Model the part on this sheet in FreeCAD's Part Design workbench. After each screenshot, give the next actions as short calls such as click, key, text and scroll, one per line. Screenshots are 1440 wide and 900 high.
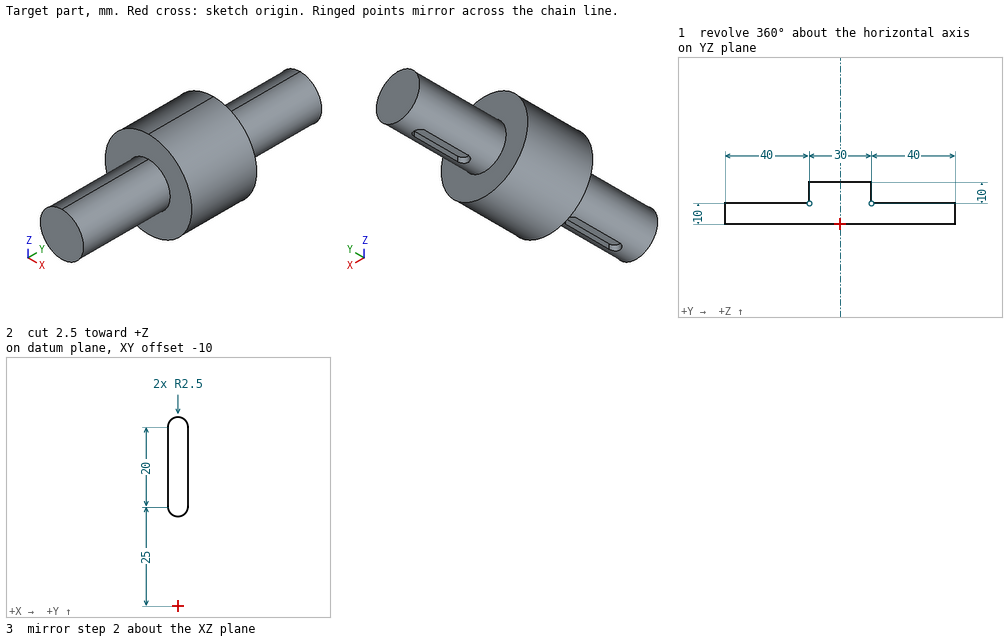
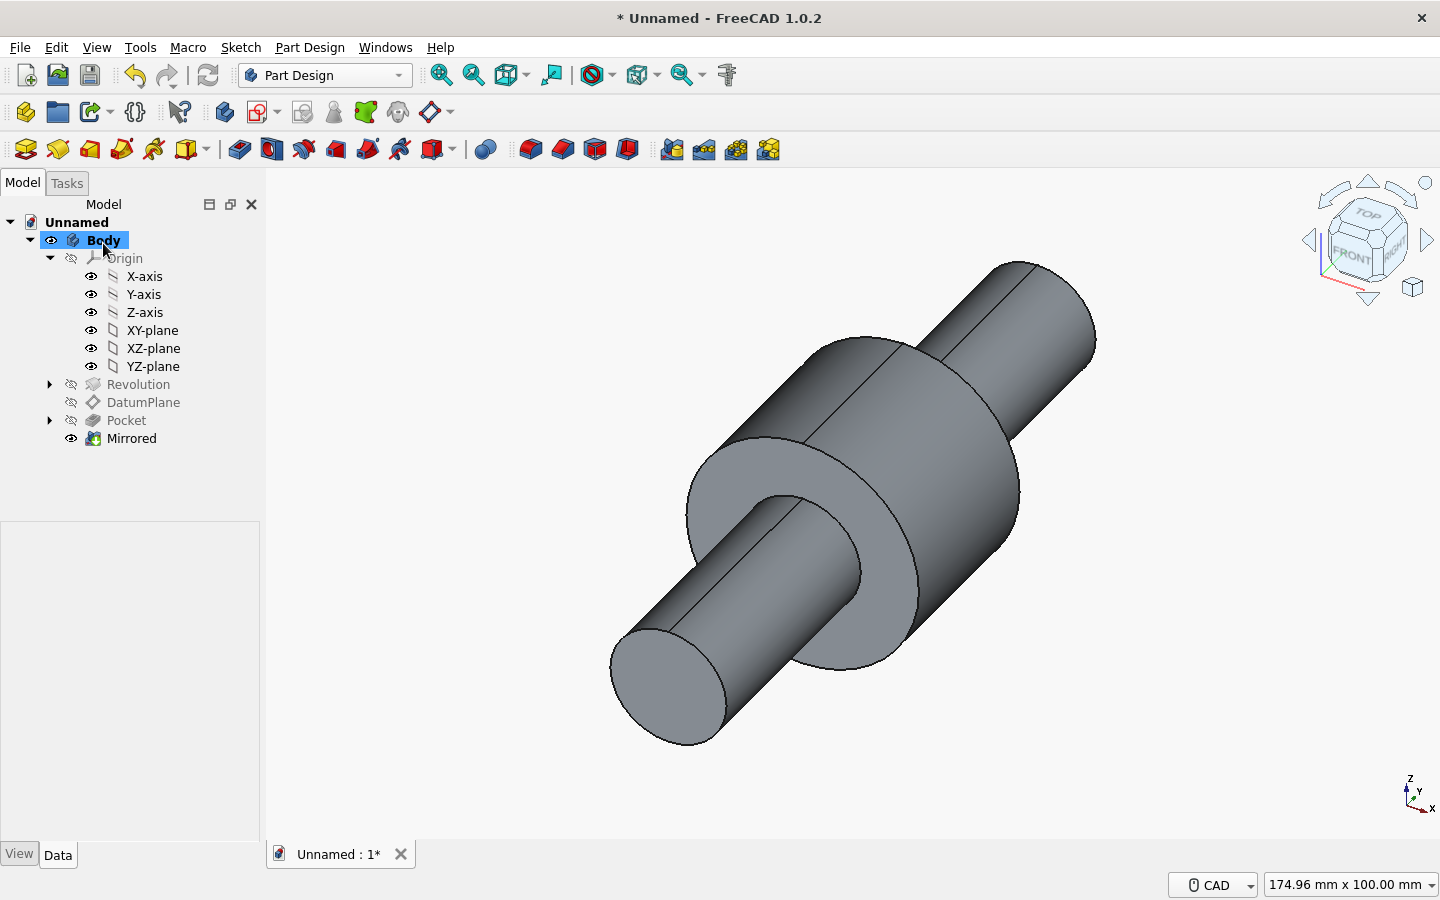
key(0)